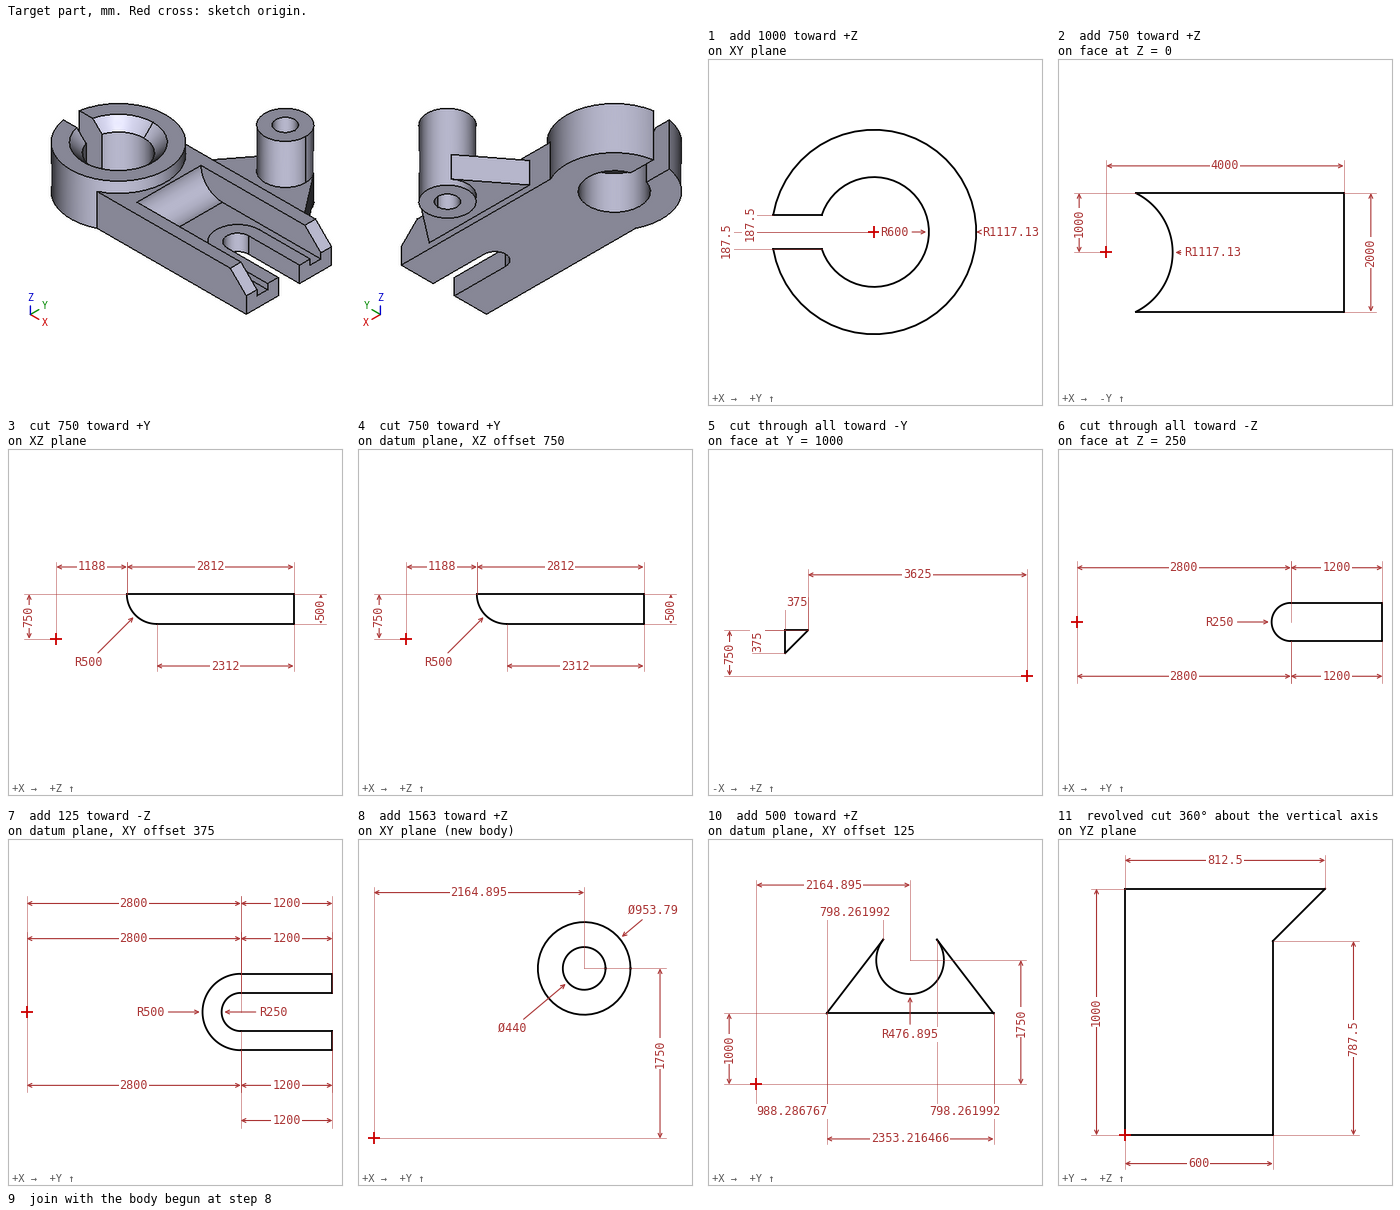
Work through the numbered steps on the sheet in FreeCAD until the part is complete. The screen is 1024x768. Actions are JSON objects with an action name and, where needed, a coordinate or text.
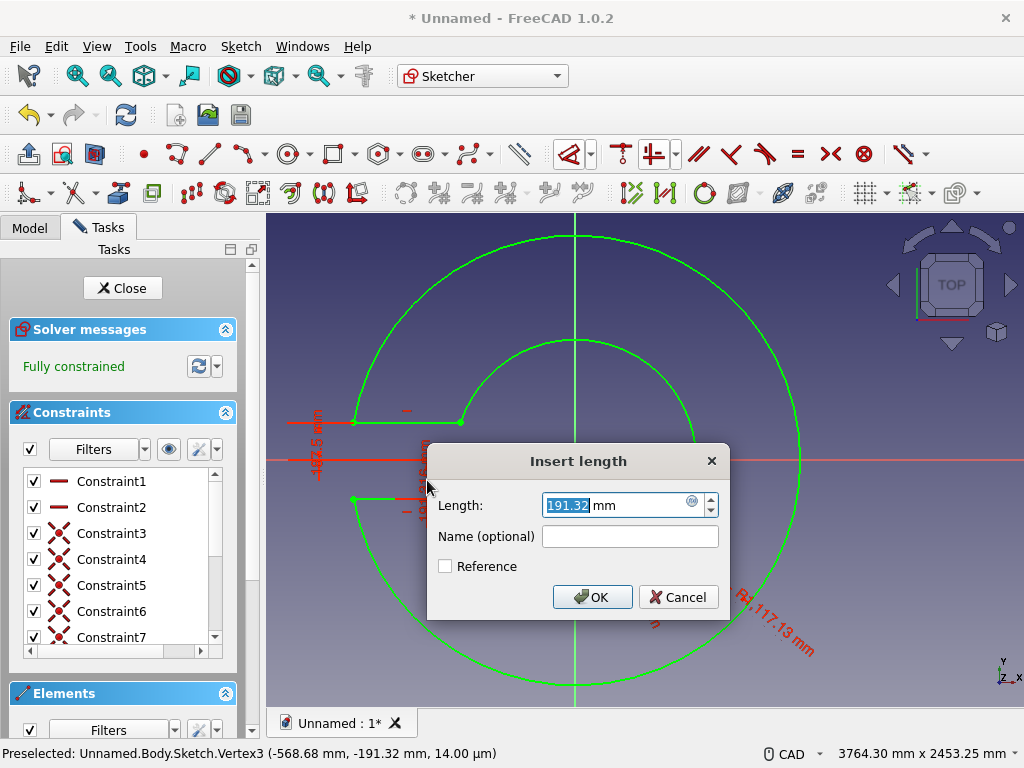
{"action": "type", "text": "187.5"}
{"action": "key", "text": "Return"}
{"action": "key", "text": "Escape"}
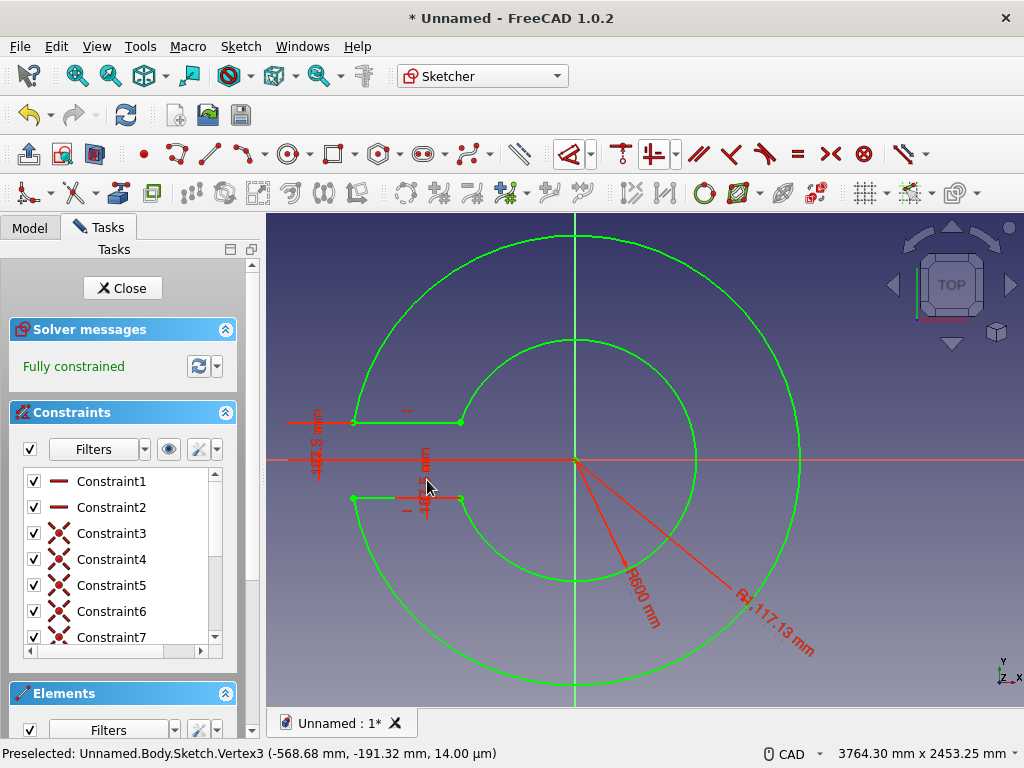
{"action": "left_click", "coordinate": [123, 288]}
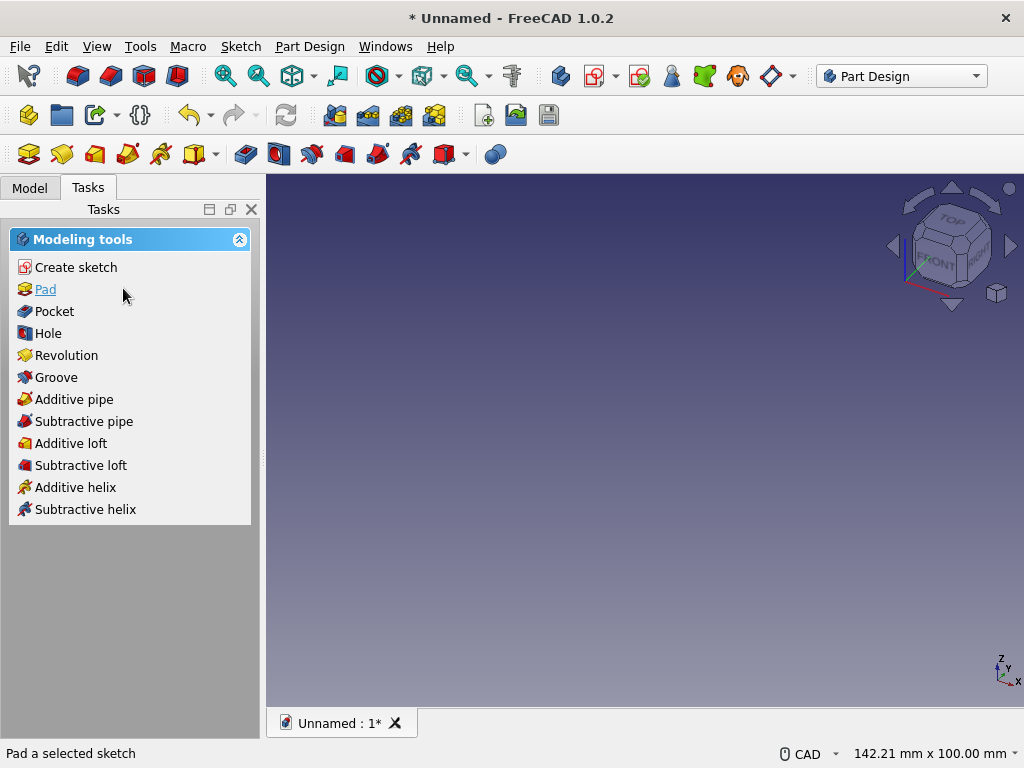
{"action": "left_click", "coordinate": [29, 154]}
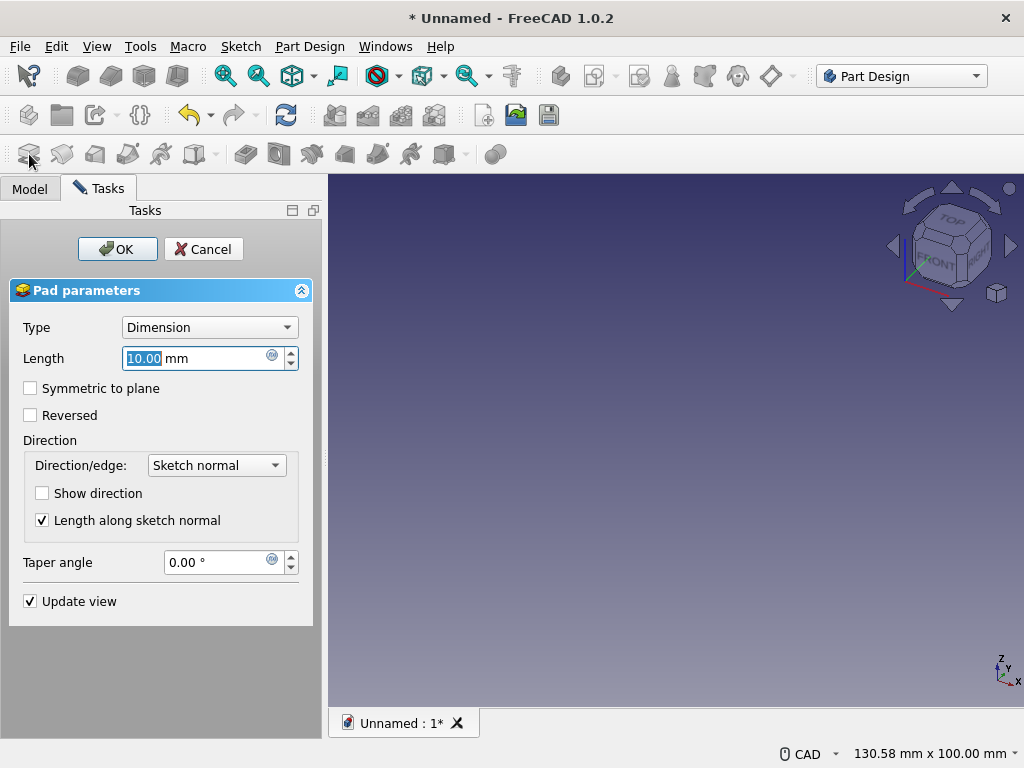
{"action": "type", "text": "1000"}
{"action": "key", "text": "Tab"}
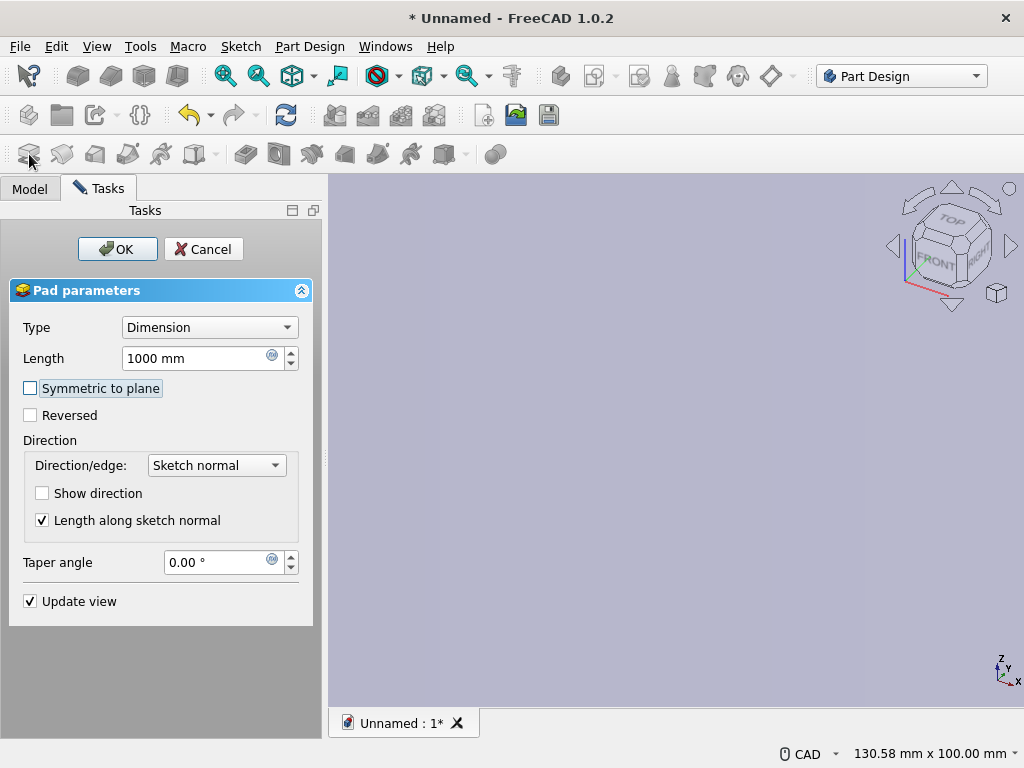
{"action": "left_click", "coordinate": [118, 249]}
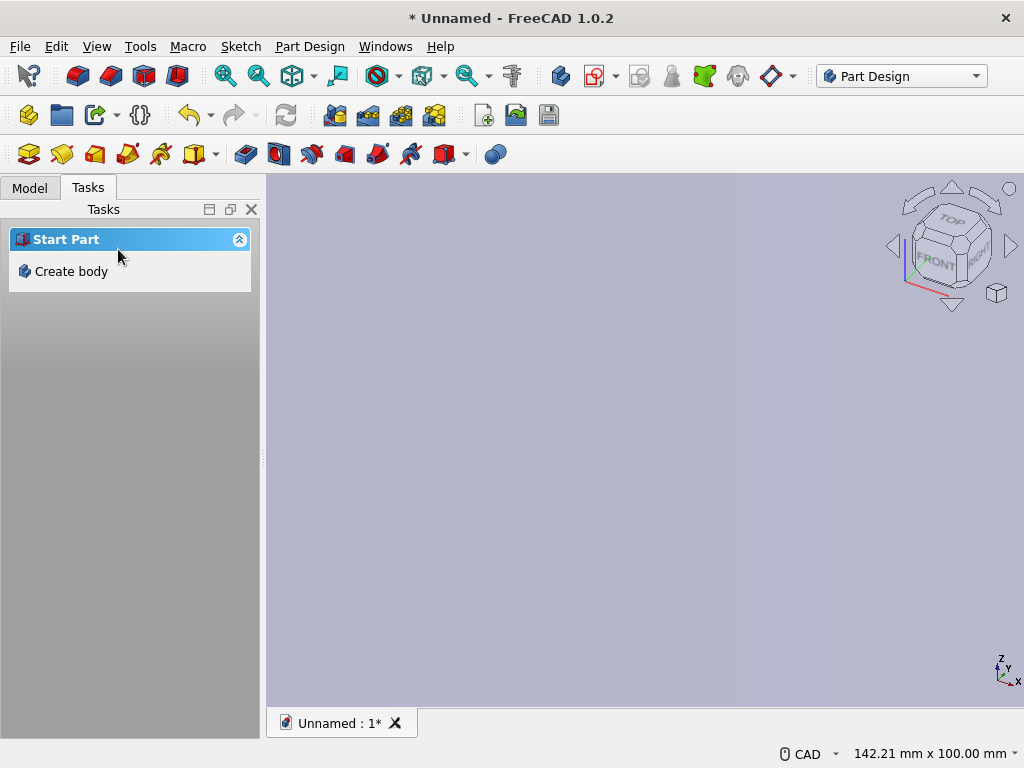
{"action": "key", "text": "v f"}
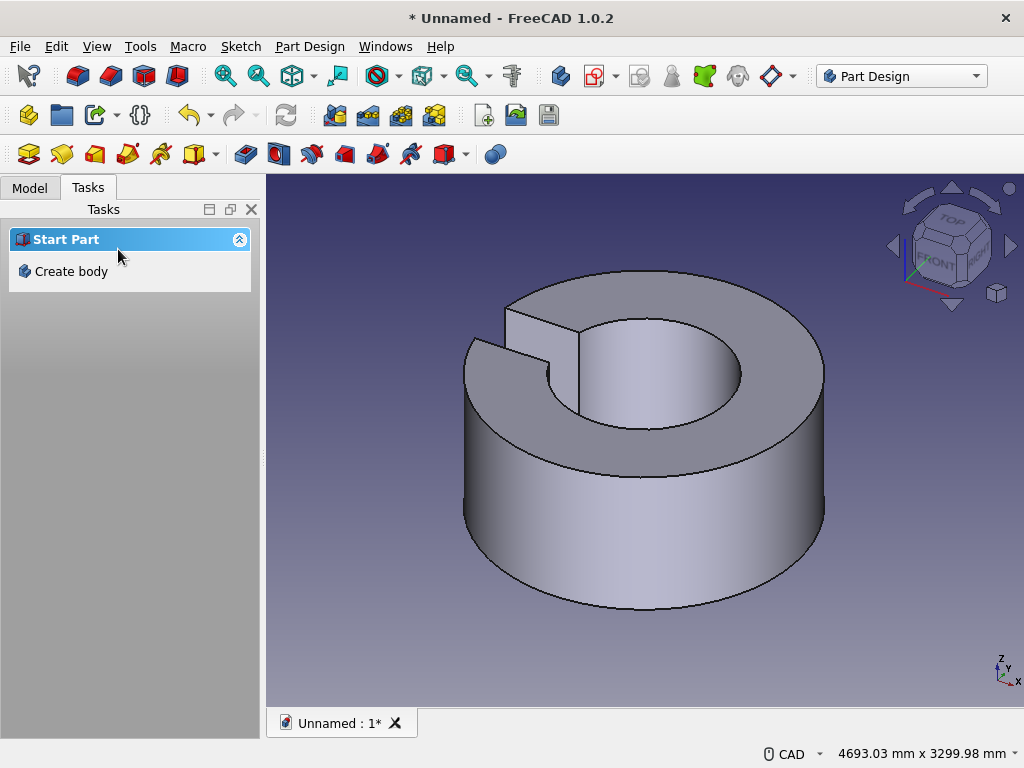
{"action": "key", "text": "5"}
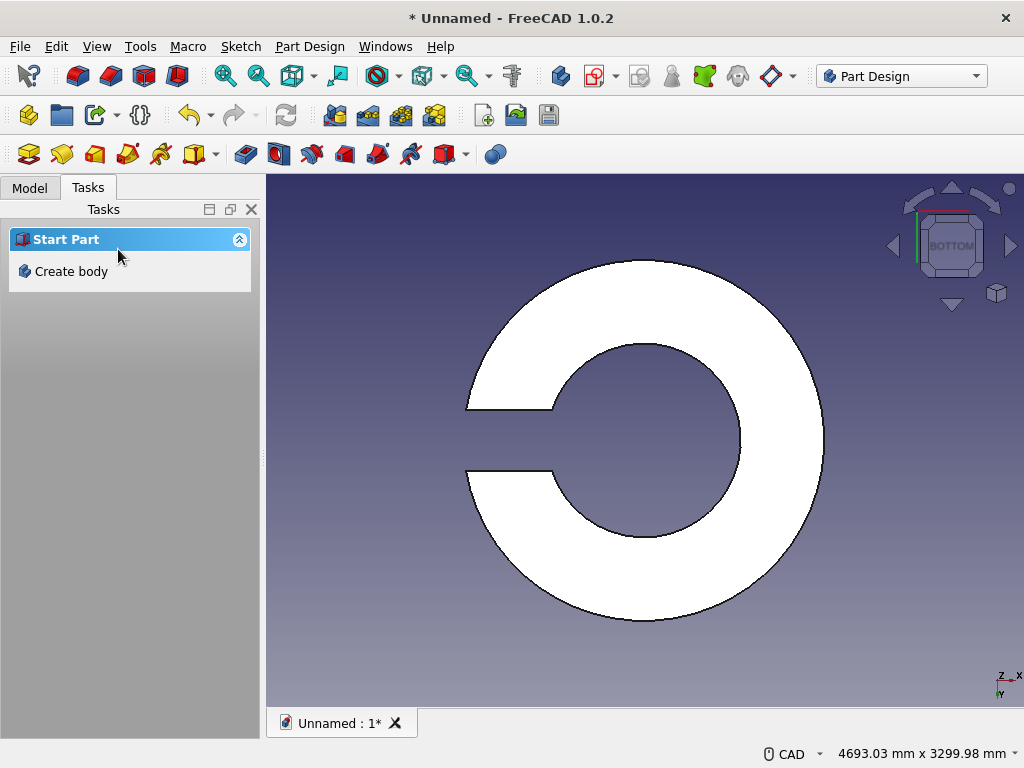
{"action": "left_click", "coordinate": [543, 543]}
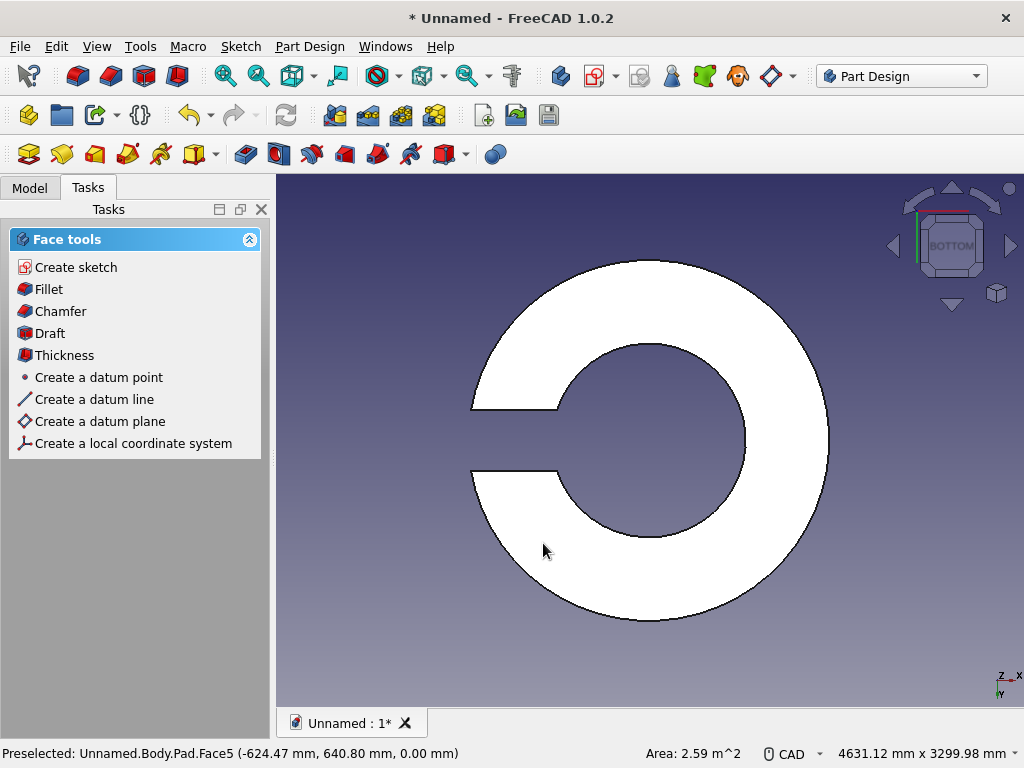
{"action": "left_click", "coordinate": [594, 76]}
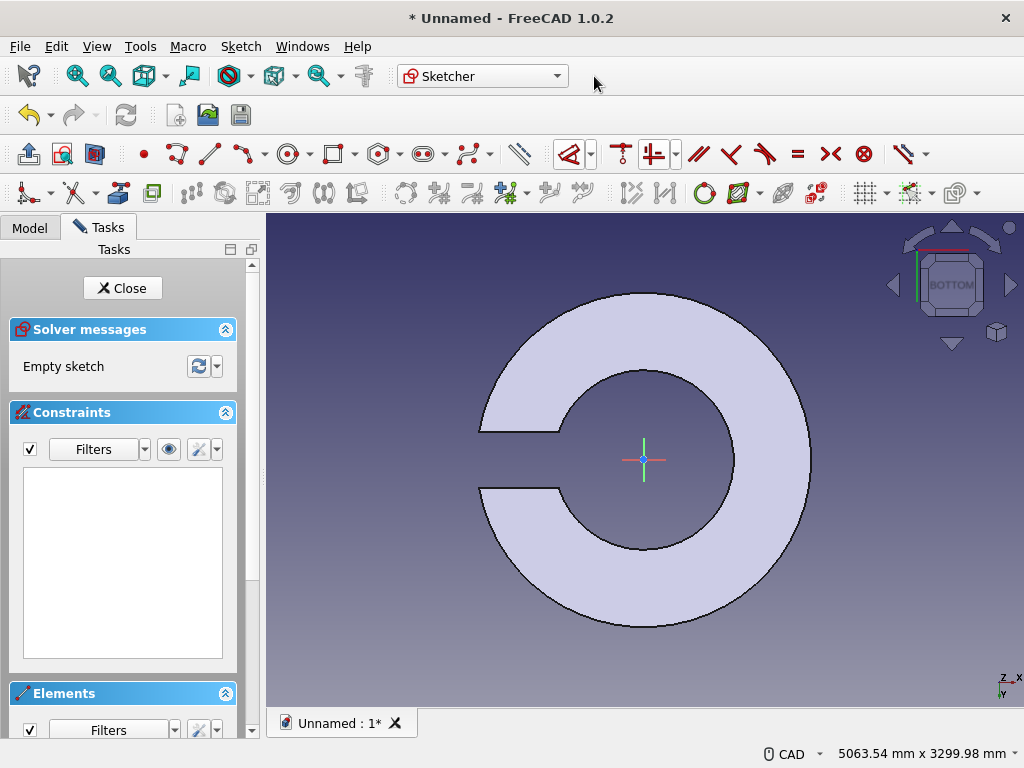
{"action": "scroll", "coordinate": [294, 460], "scroll_direction": "down", "scroll_amount": 3}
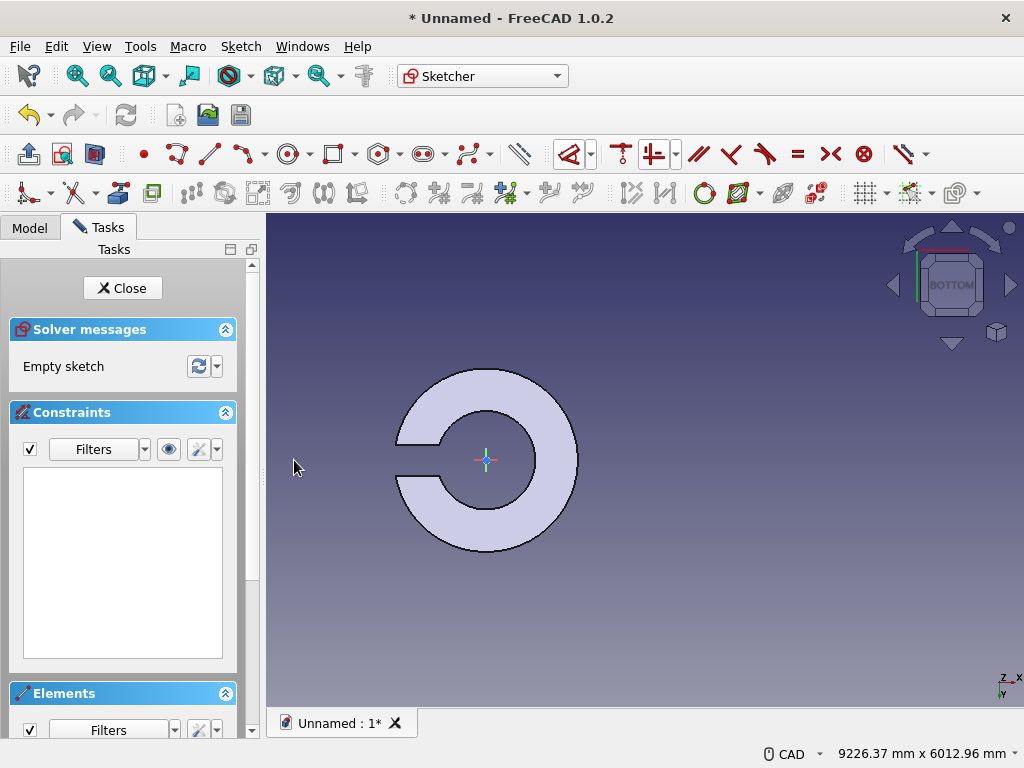
{"action": "left_click", "coordinate": [177, 154]}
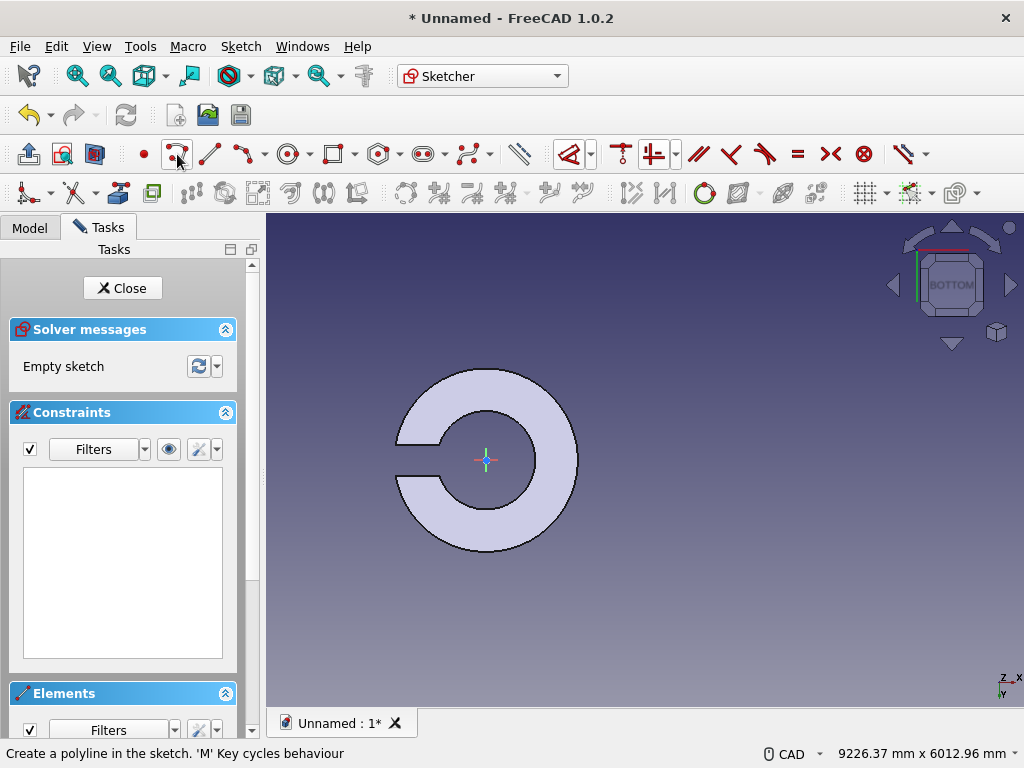
{"action": "left_click", "coordinate": [527, 378]}
{"action": "left_click", "coordinate": [815, 378]}
{"action": "left_click", "coordinate": [815, 542]}
{"action": "left_click", "coordinate": [527, 542]}
{"action": "right_click", "coordinate": [527, 542]}